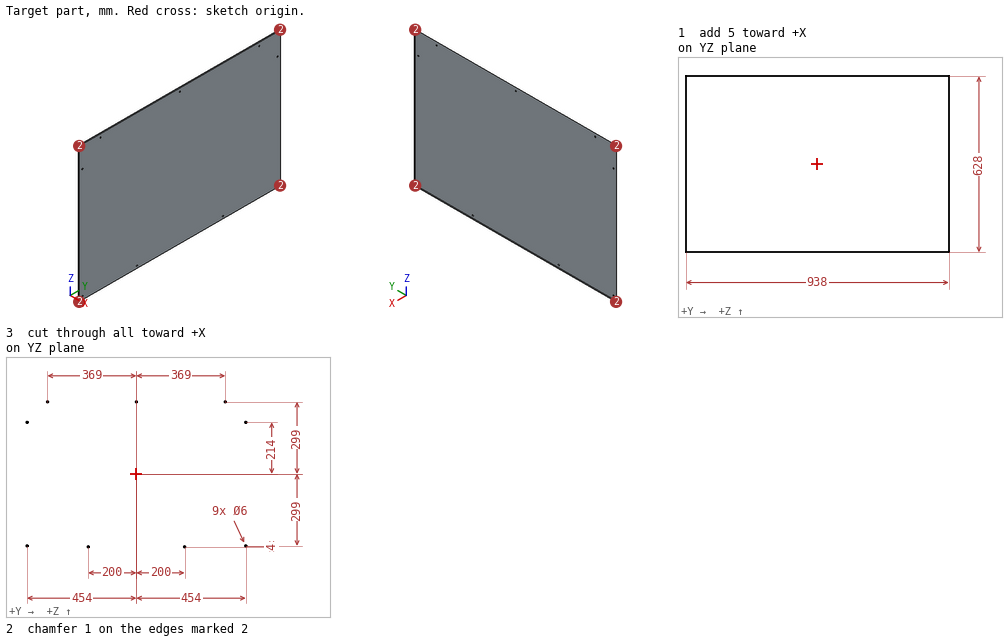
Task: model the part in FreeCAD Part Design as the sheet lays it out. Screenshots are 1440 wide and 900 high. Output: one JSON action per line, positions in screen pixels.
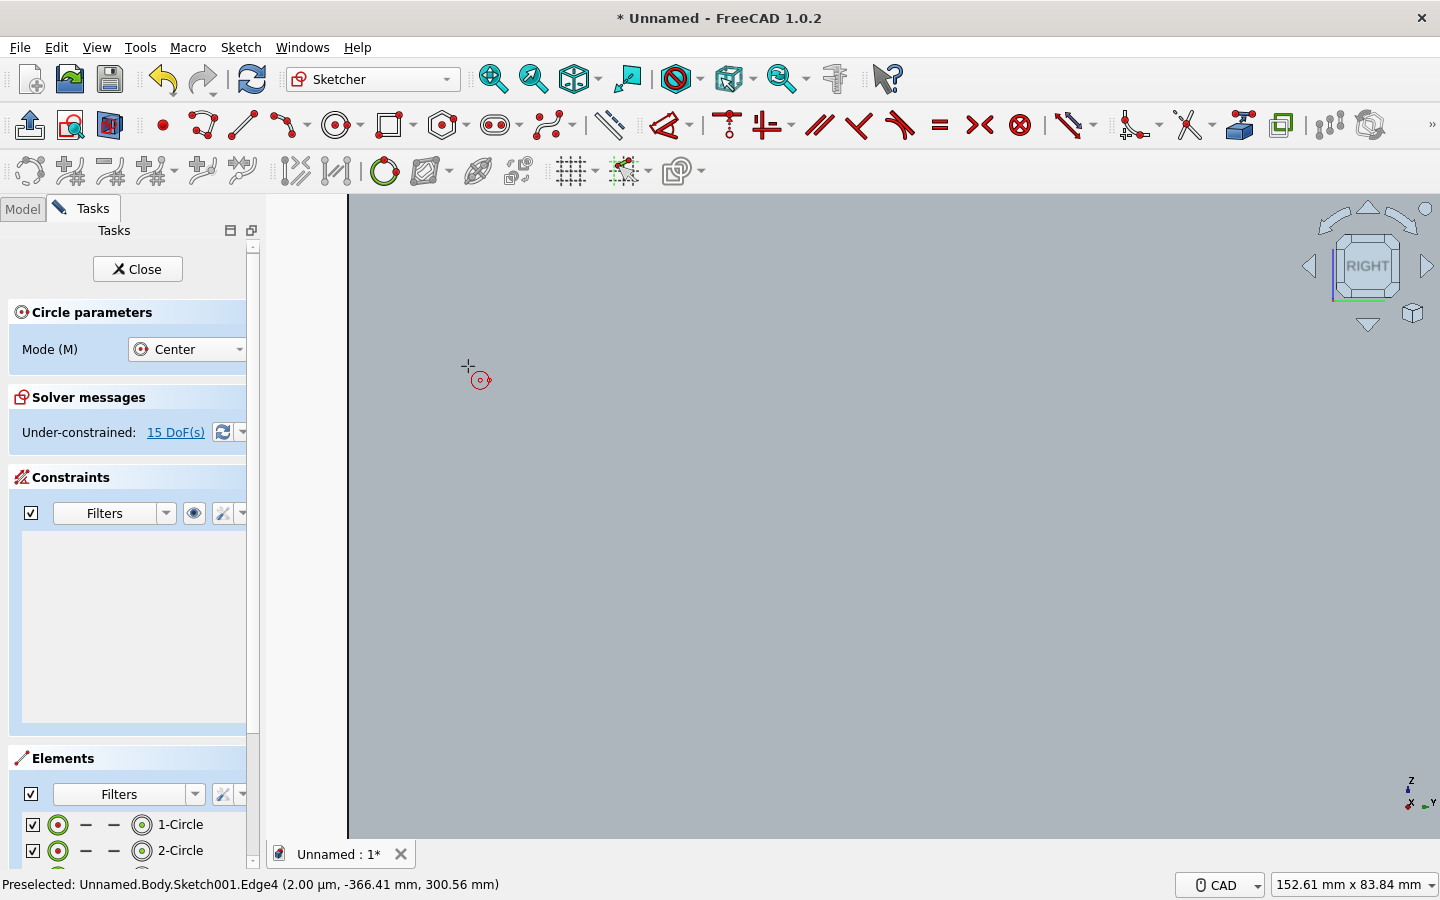
{"action": "scroll", "coordinate": [468, 366], "scroll_direction": "down", "scroll_amount": 12}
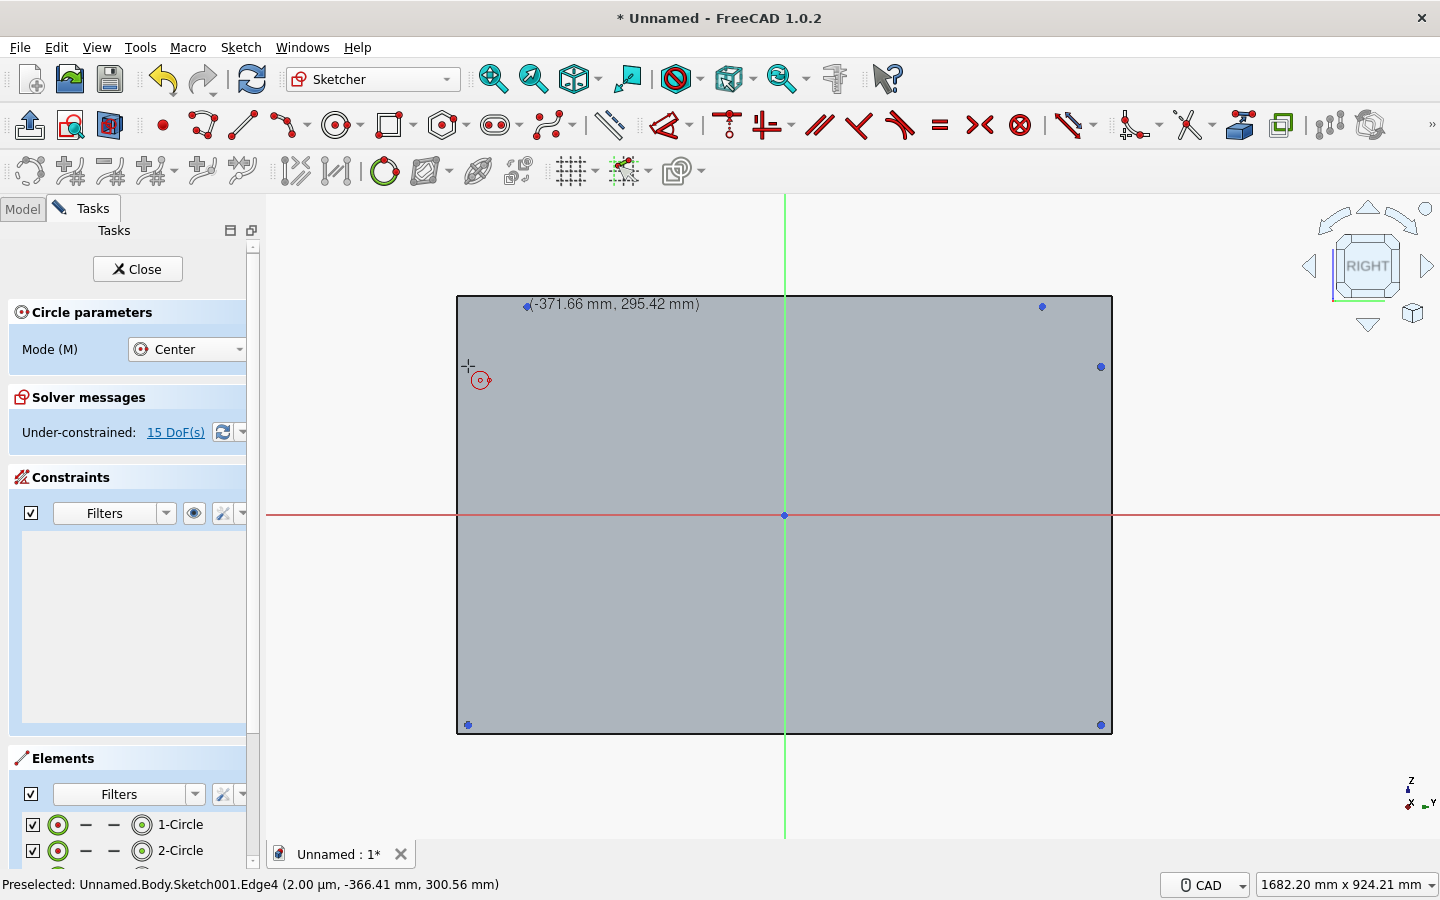
{"action": "left_click", "coordinate": [468, 366]}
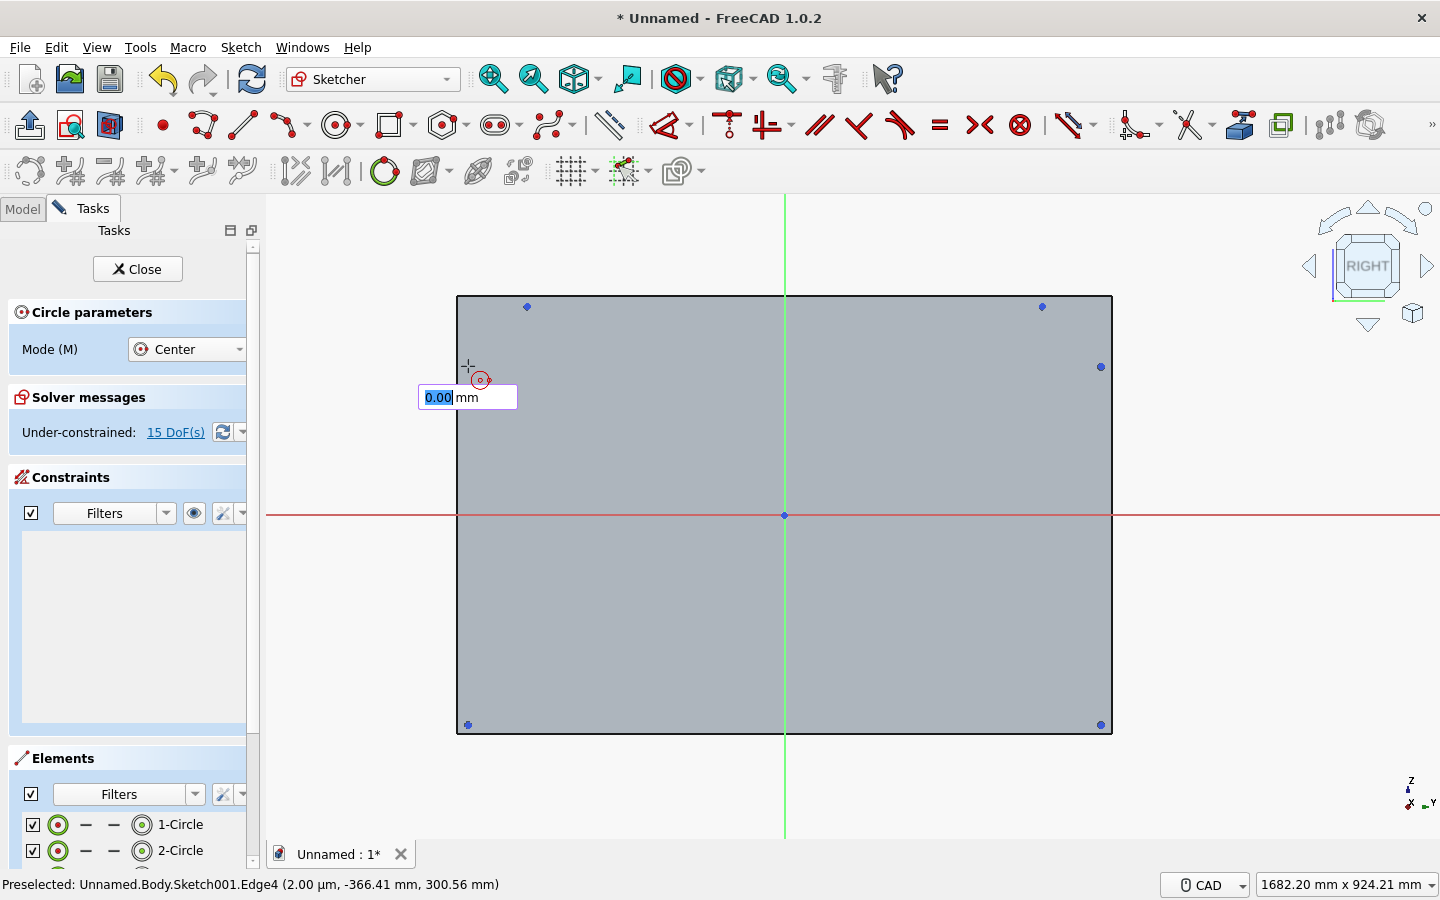
{"action": "scroll", "coordinate": [469, 364], "scroll_direction": "up", "scroll_amount": 11}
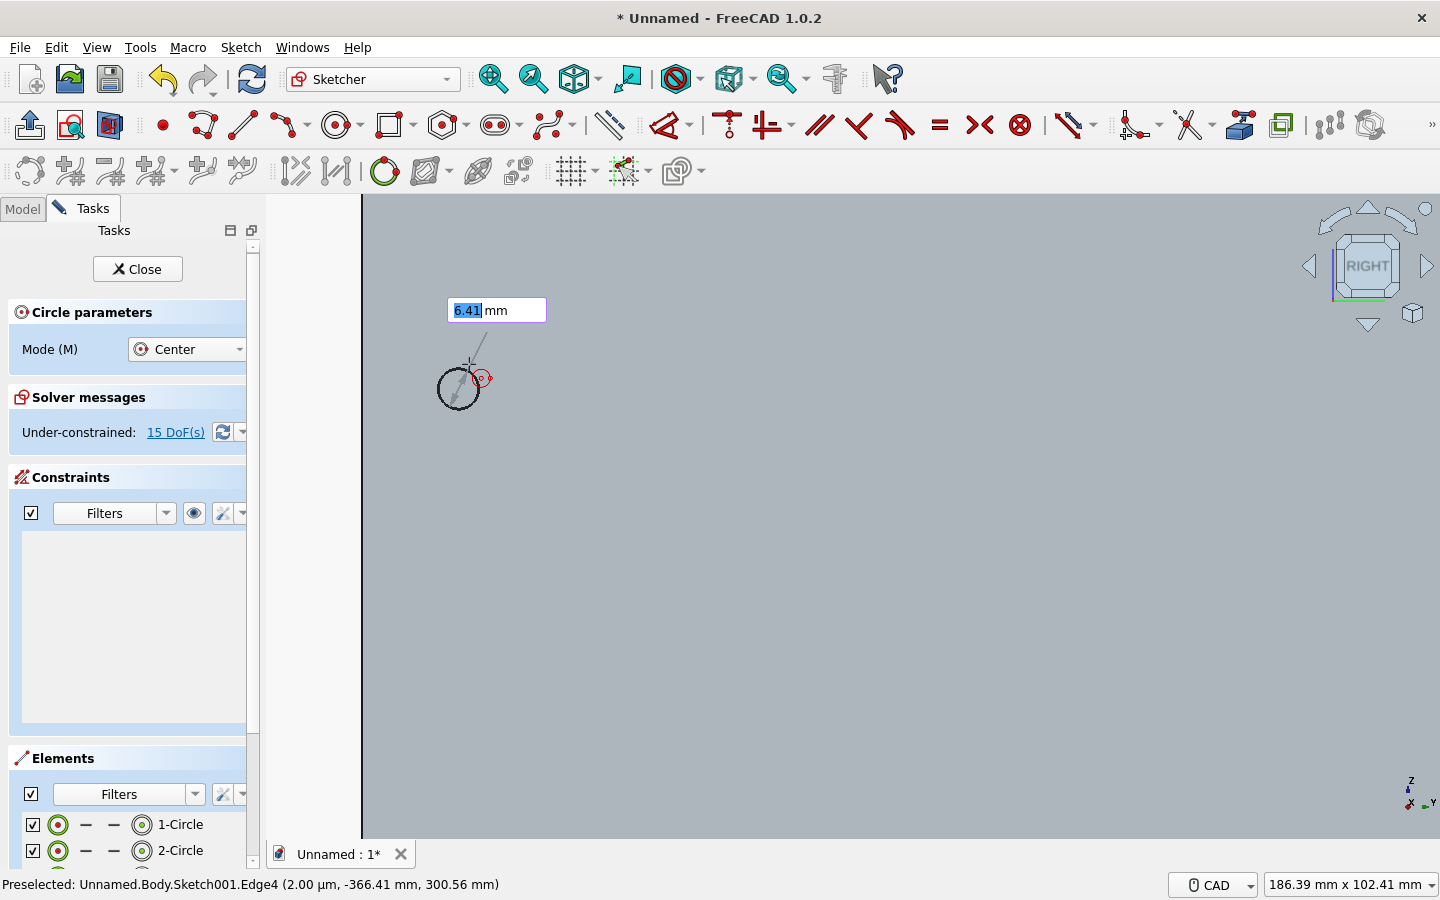
{"action": "left_click", "coordinate": [470, 363]}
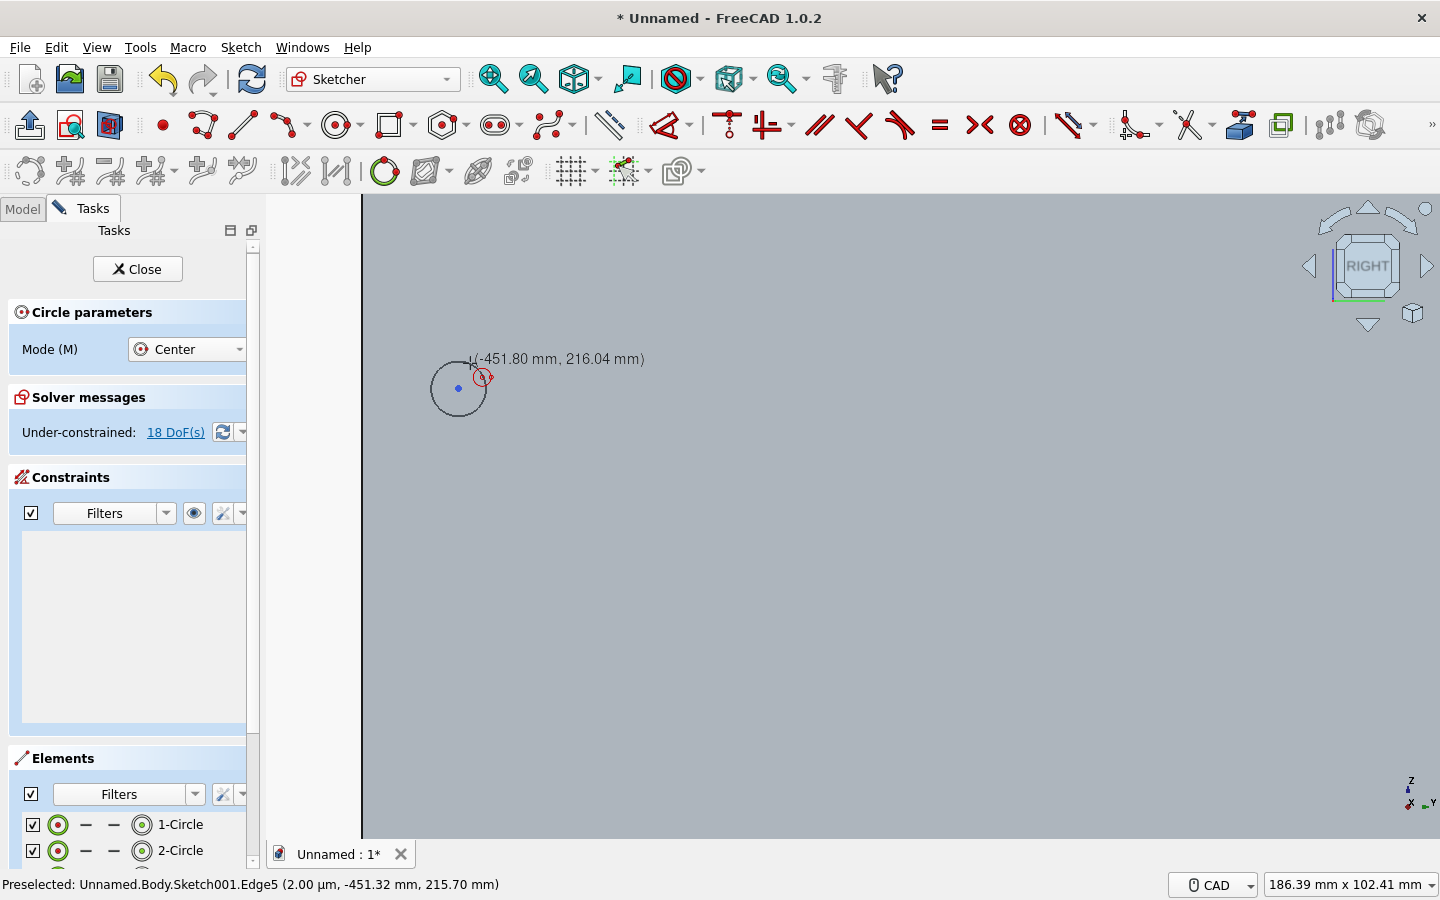
{"action": "scroll", "coordinate": [469, 364], "scroll_direction": "down", "scroll_amount": 11}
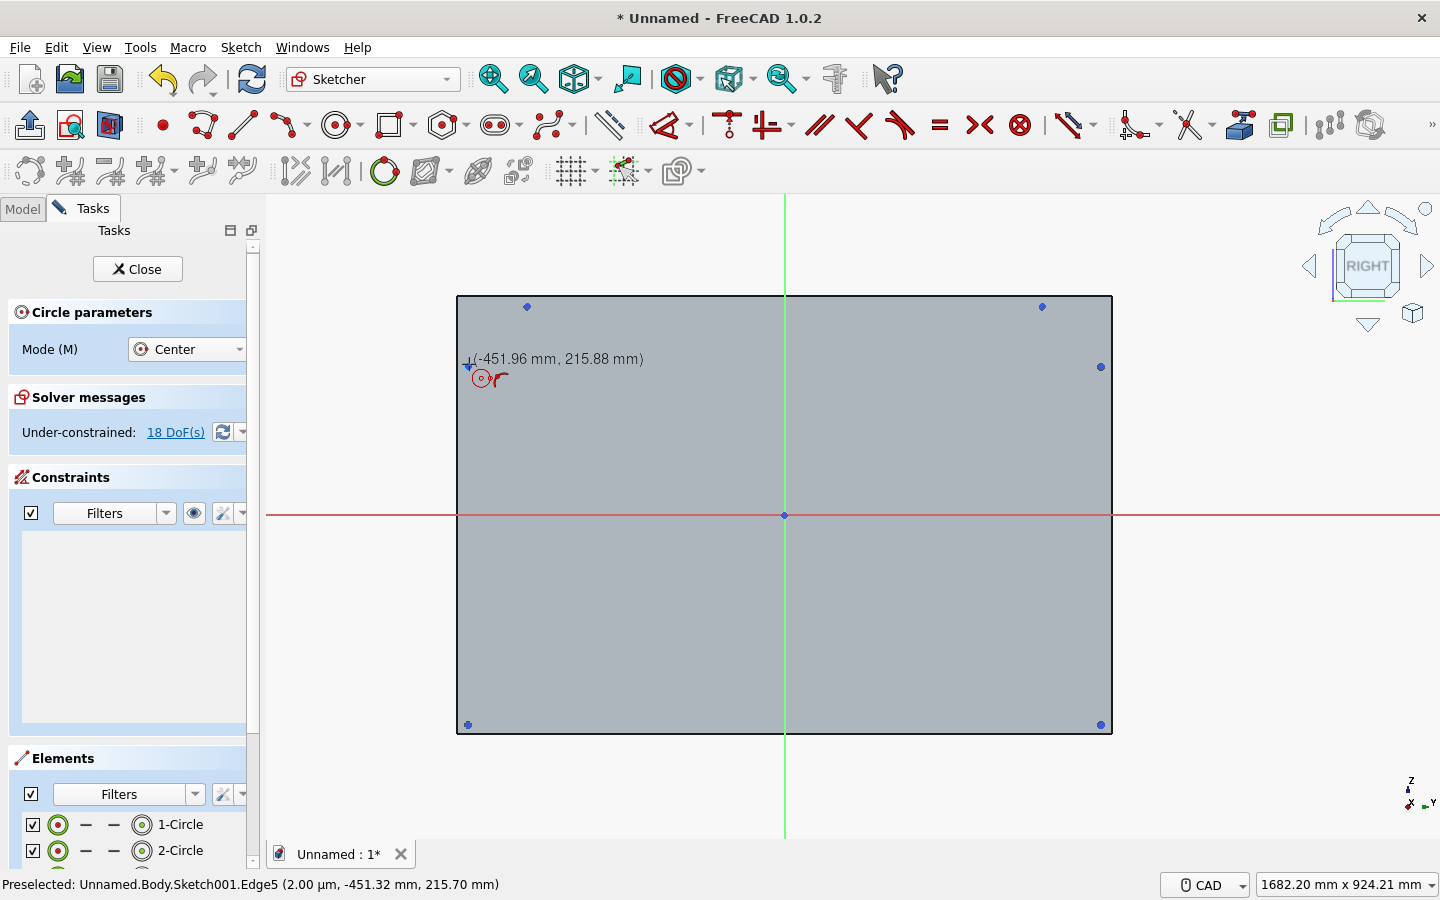
{"action": "scroll", "coordinate": [785, 306], "scroll_direction": "up", "scroll_amount": 12}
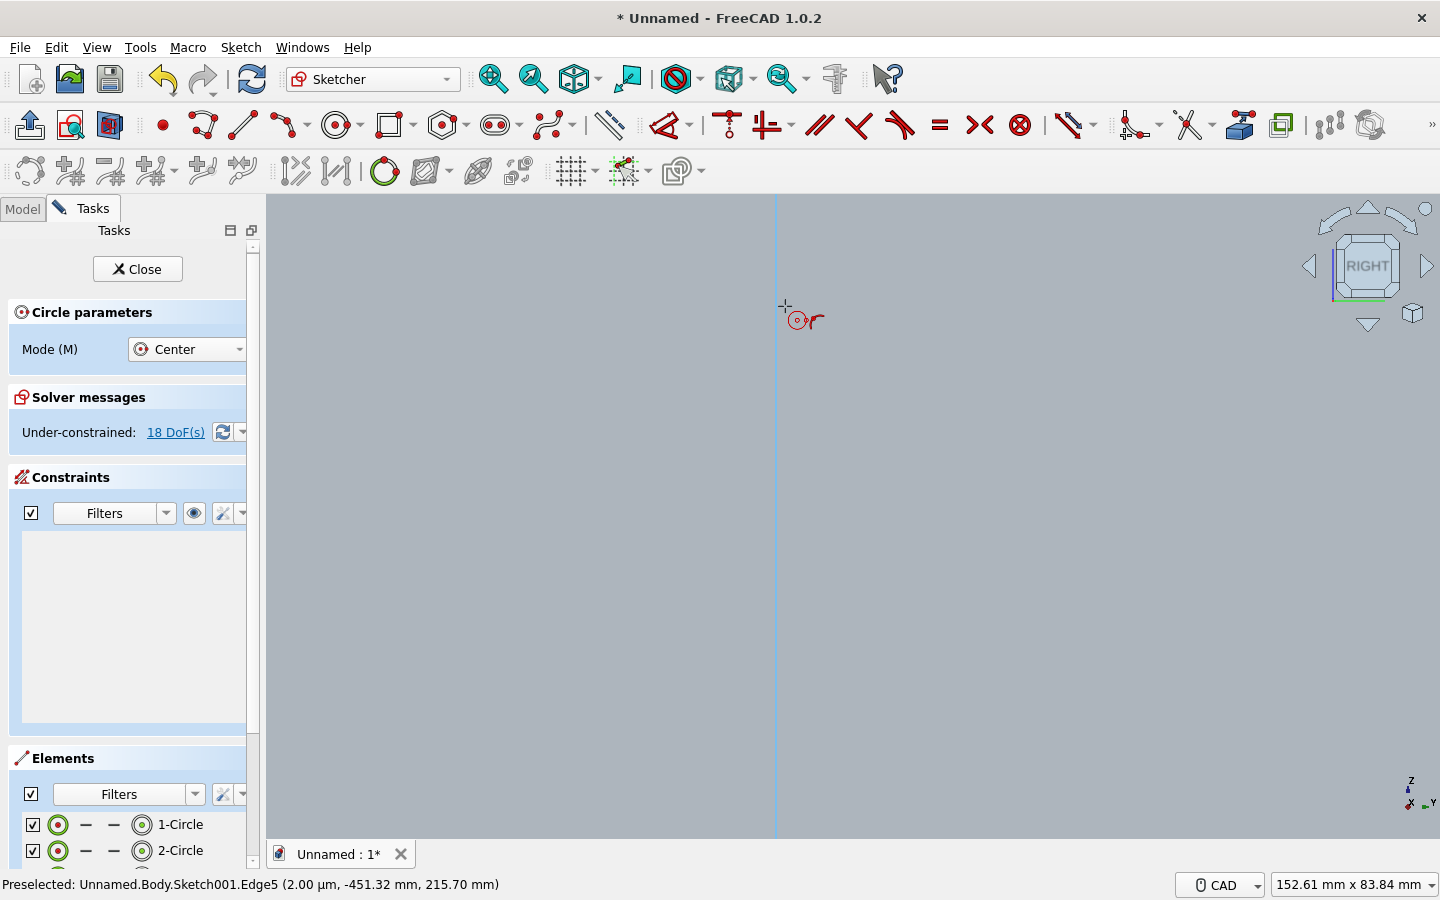
{"action": "scroll", "coordinate": [785, 306], "scroll_direction": "down", "scroll_amount": 12}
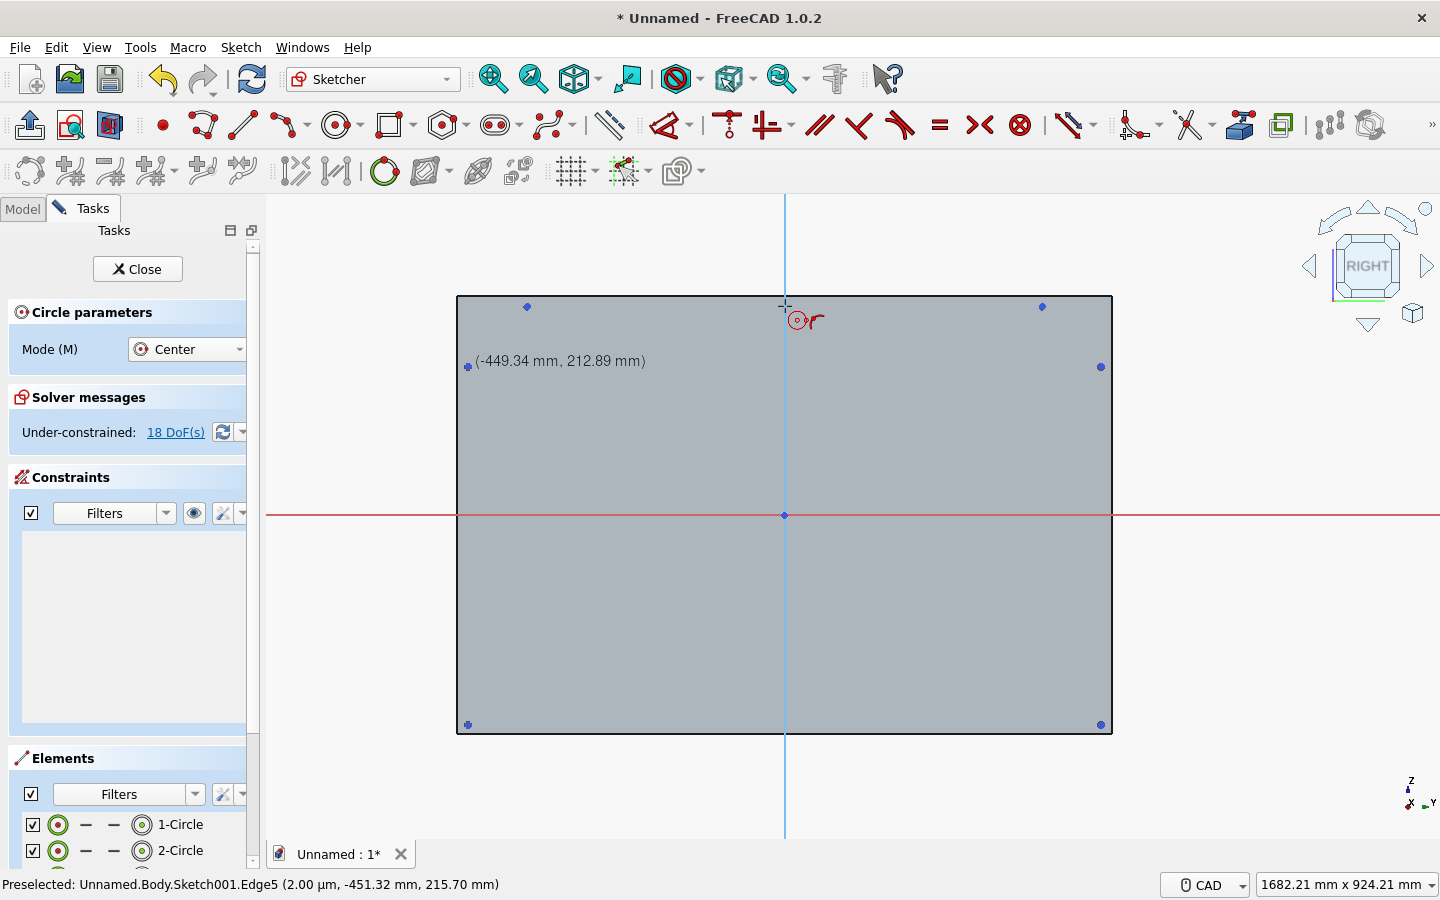
{"action": "left_click", "coordinate": [785, 306]}